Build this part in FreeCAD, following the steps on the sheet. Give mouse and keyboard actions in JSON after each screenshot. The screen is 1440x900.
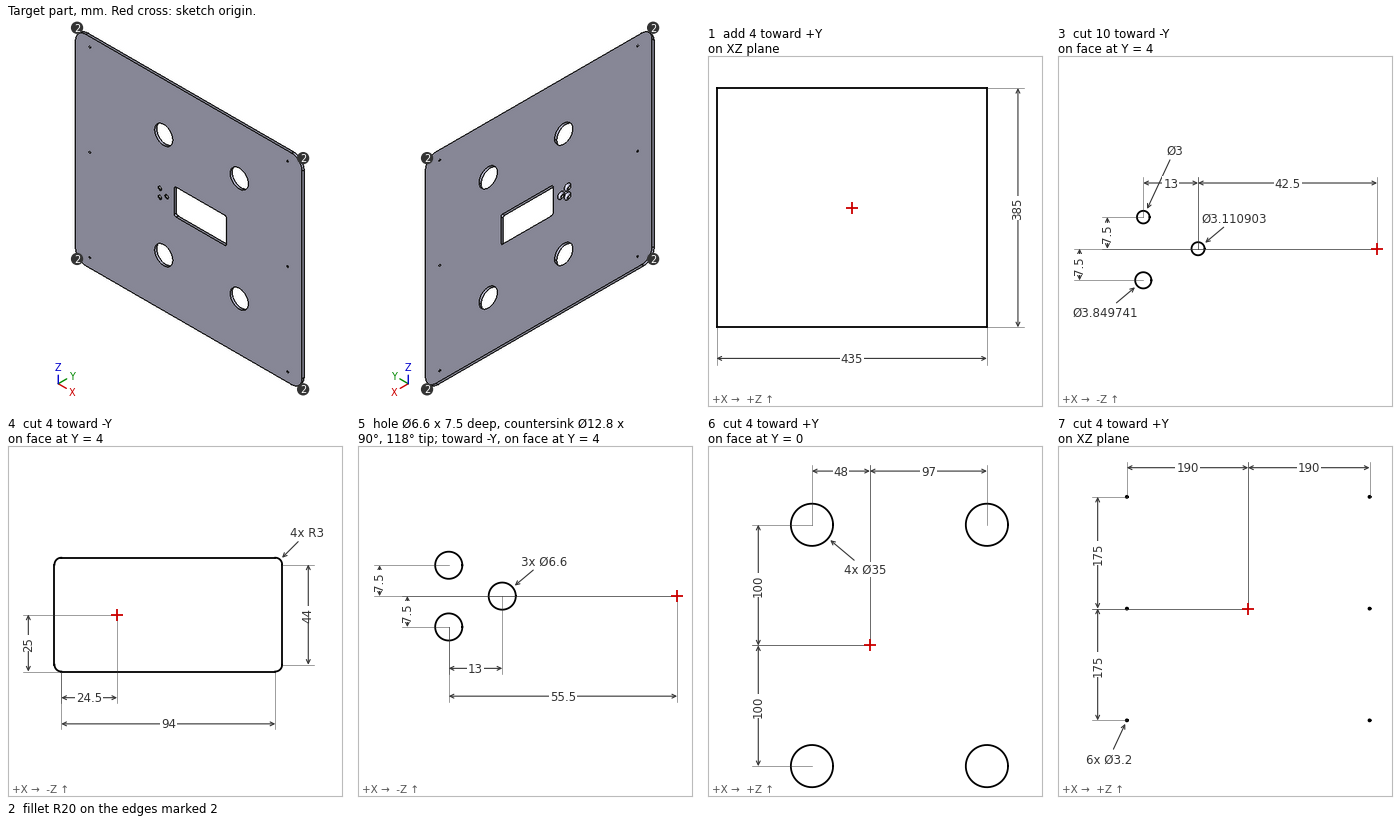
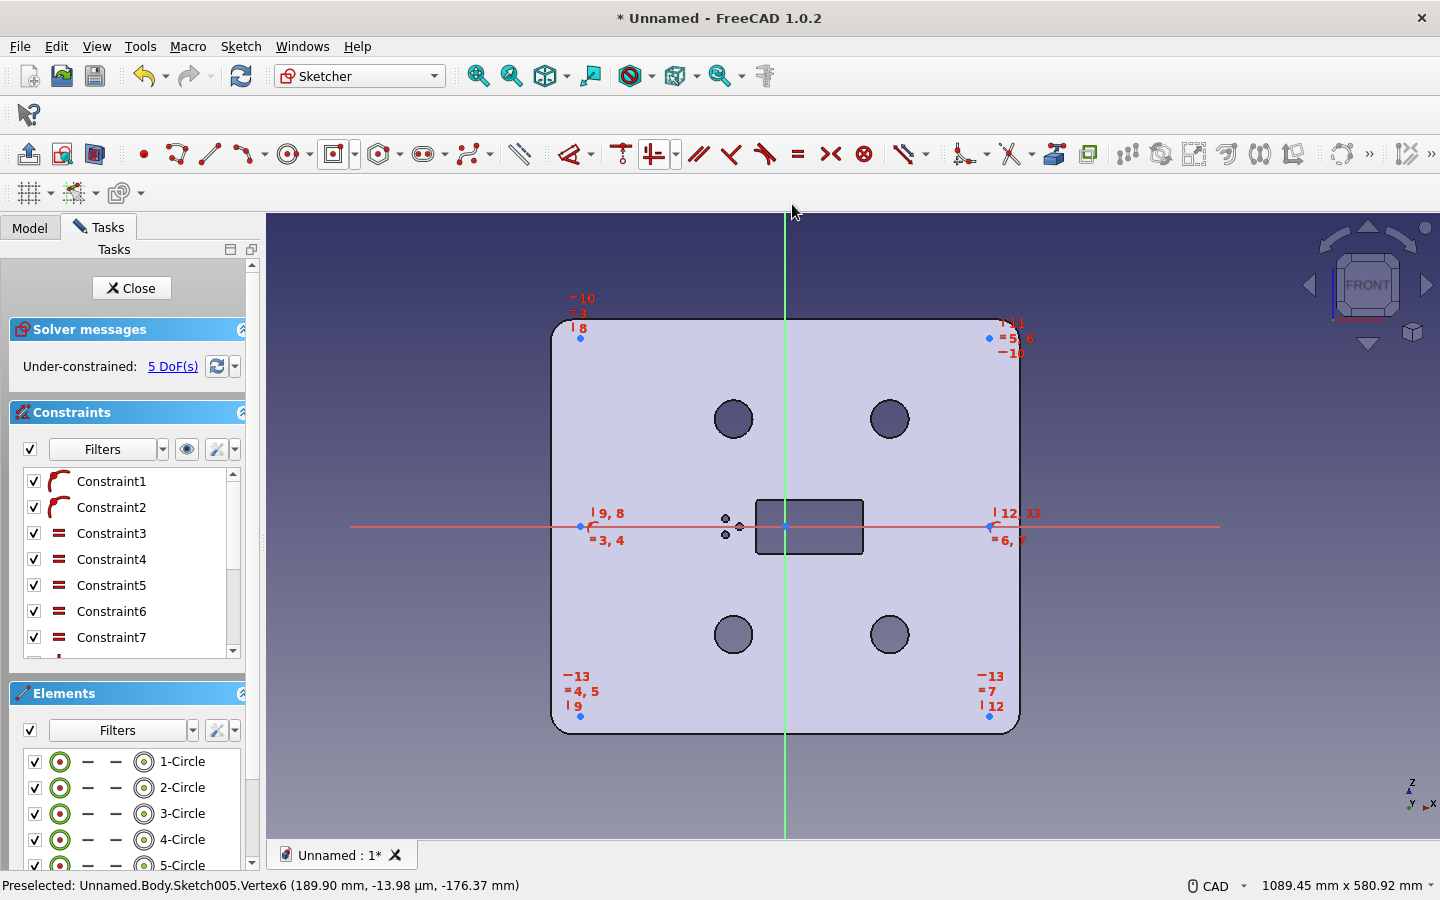
{"action": "left_click", "coordinate": [568, 154]}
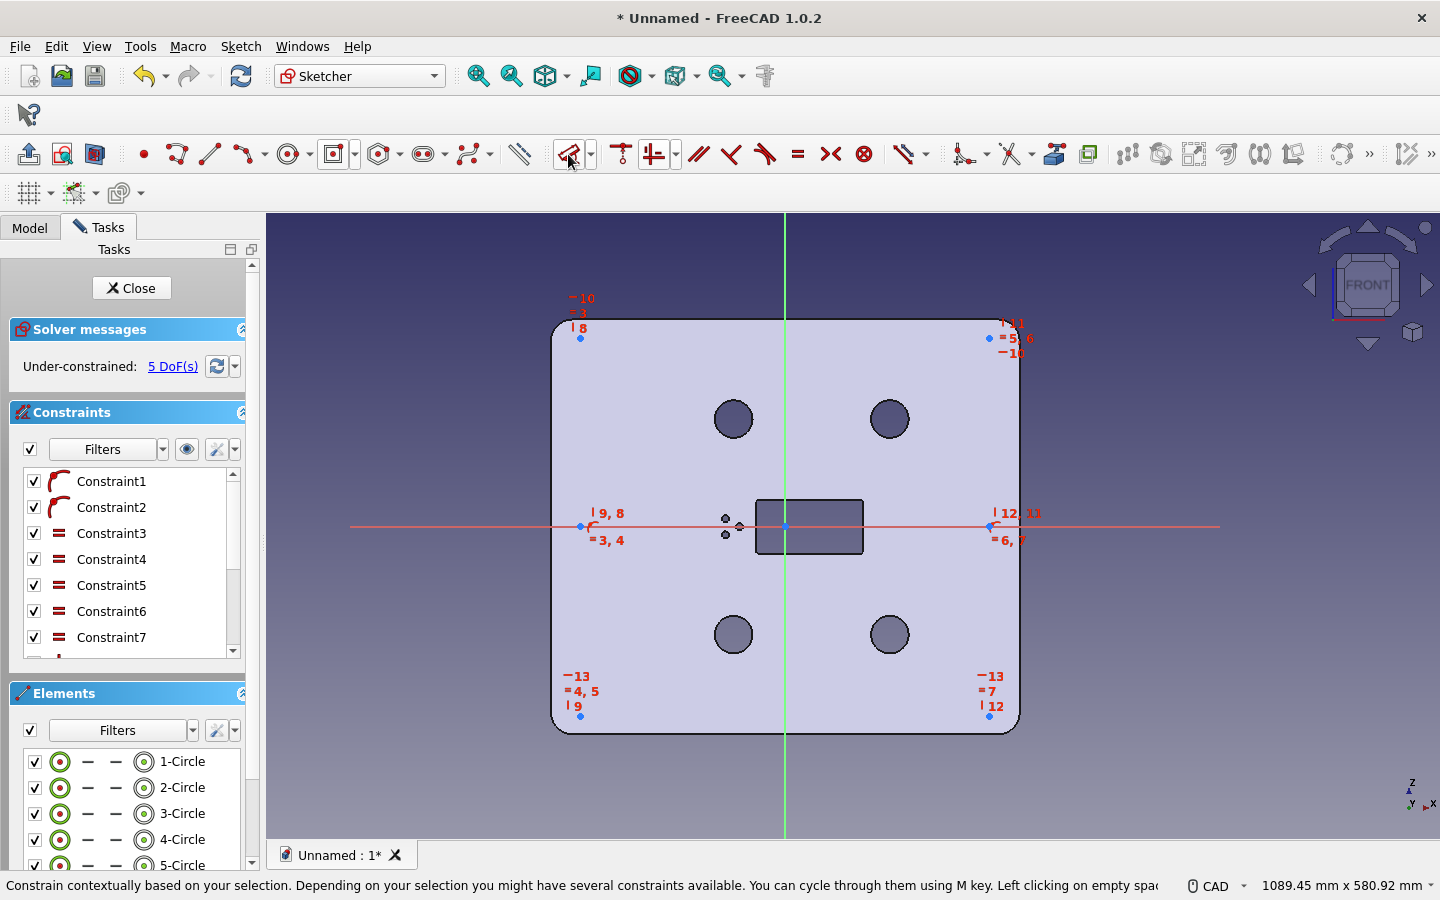
{"action": "scroll", "coordinate": [582, 337], "scroll_direction": "up", "scroll_amount": 13}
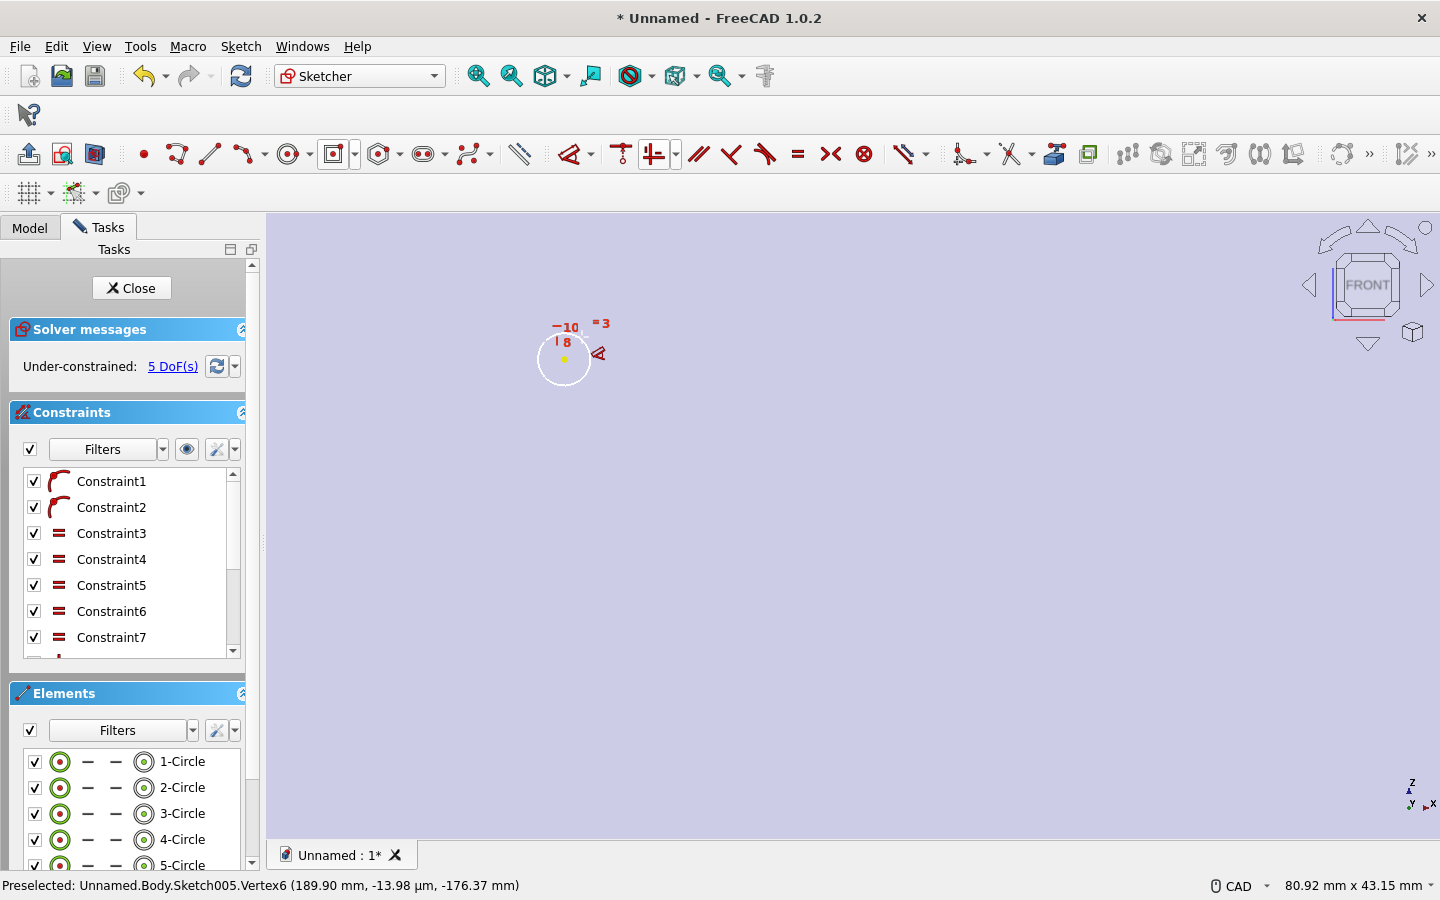
{"action": "left_click", "coordinate": [583, 341]}
{"action": "left_click", "coordinate": [606, 319]}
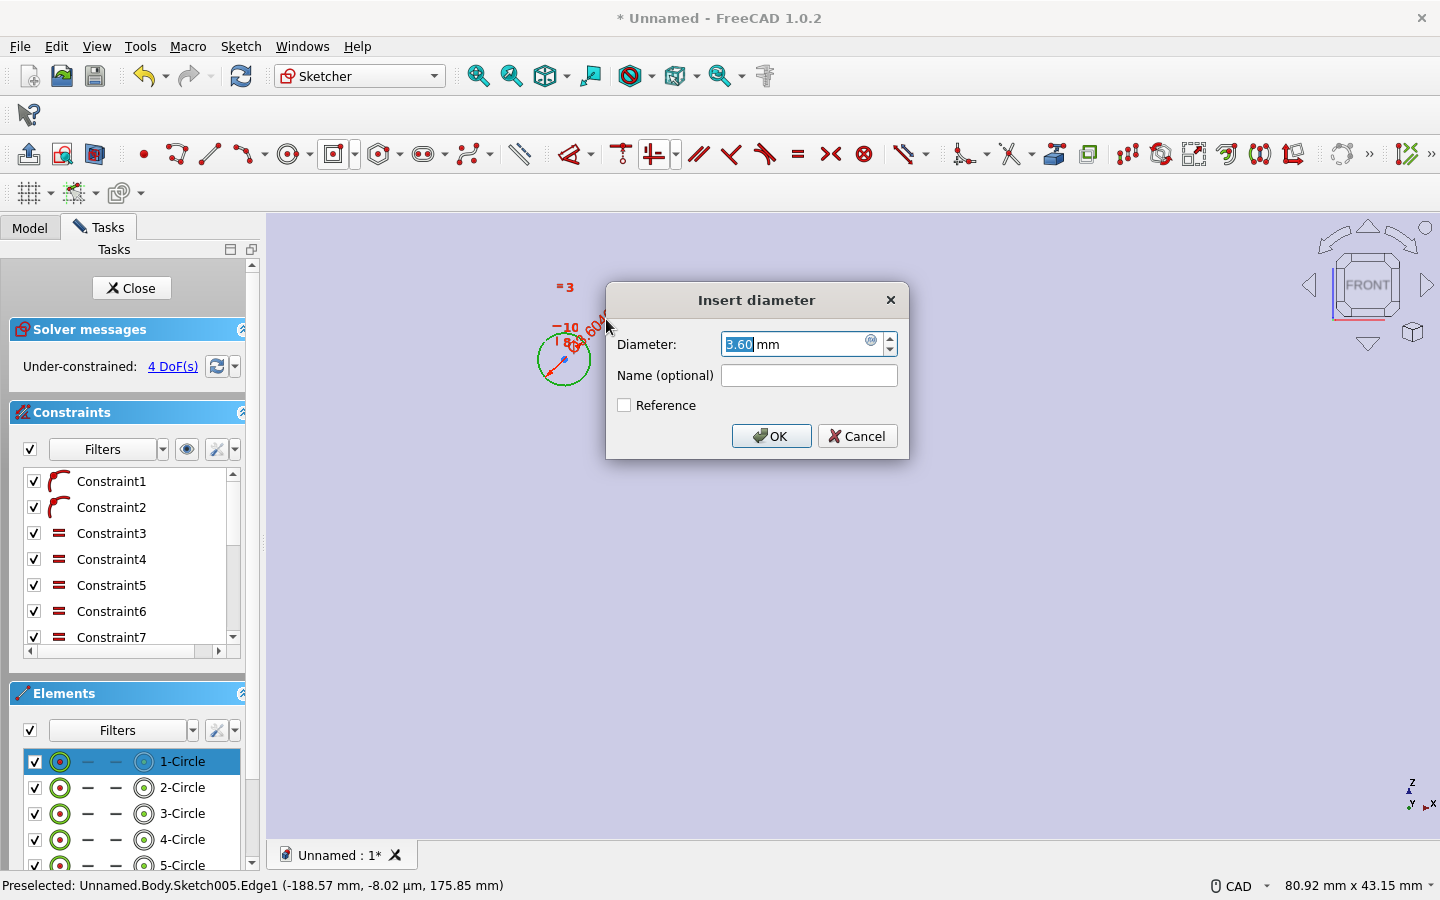
{"action": "type", "text": "3.2"}
{"action": "key", "text": "Return"}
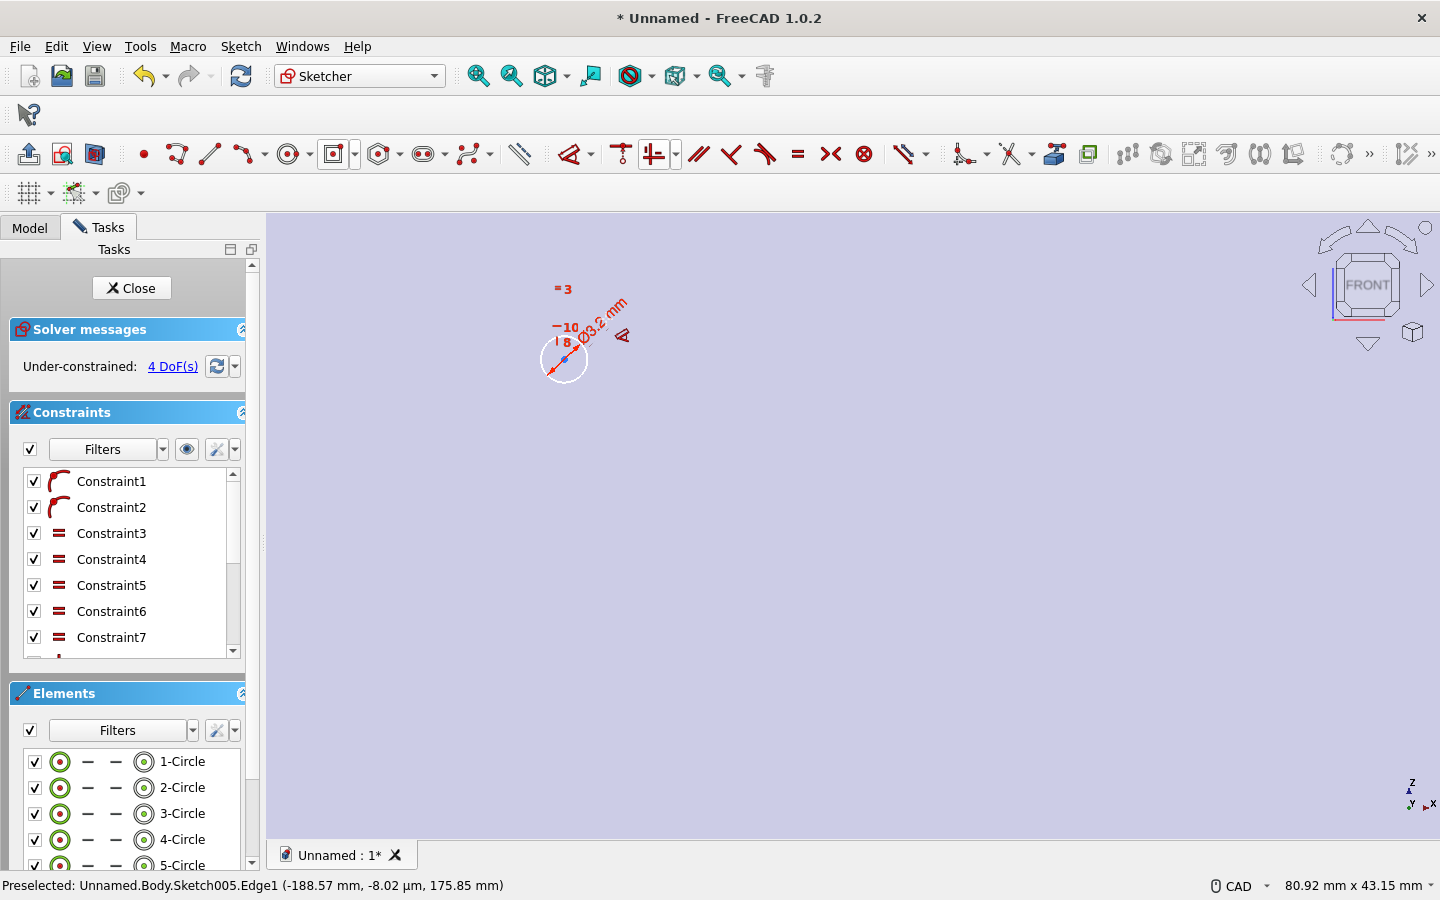
{"action": "scroll", "coordinate": [581, 336], "scroll_direction": "down", "scroll_amount": 13}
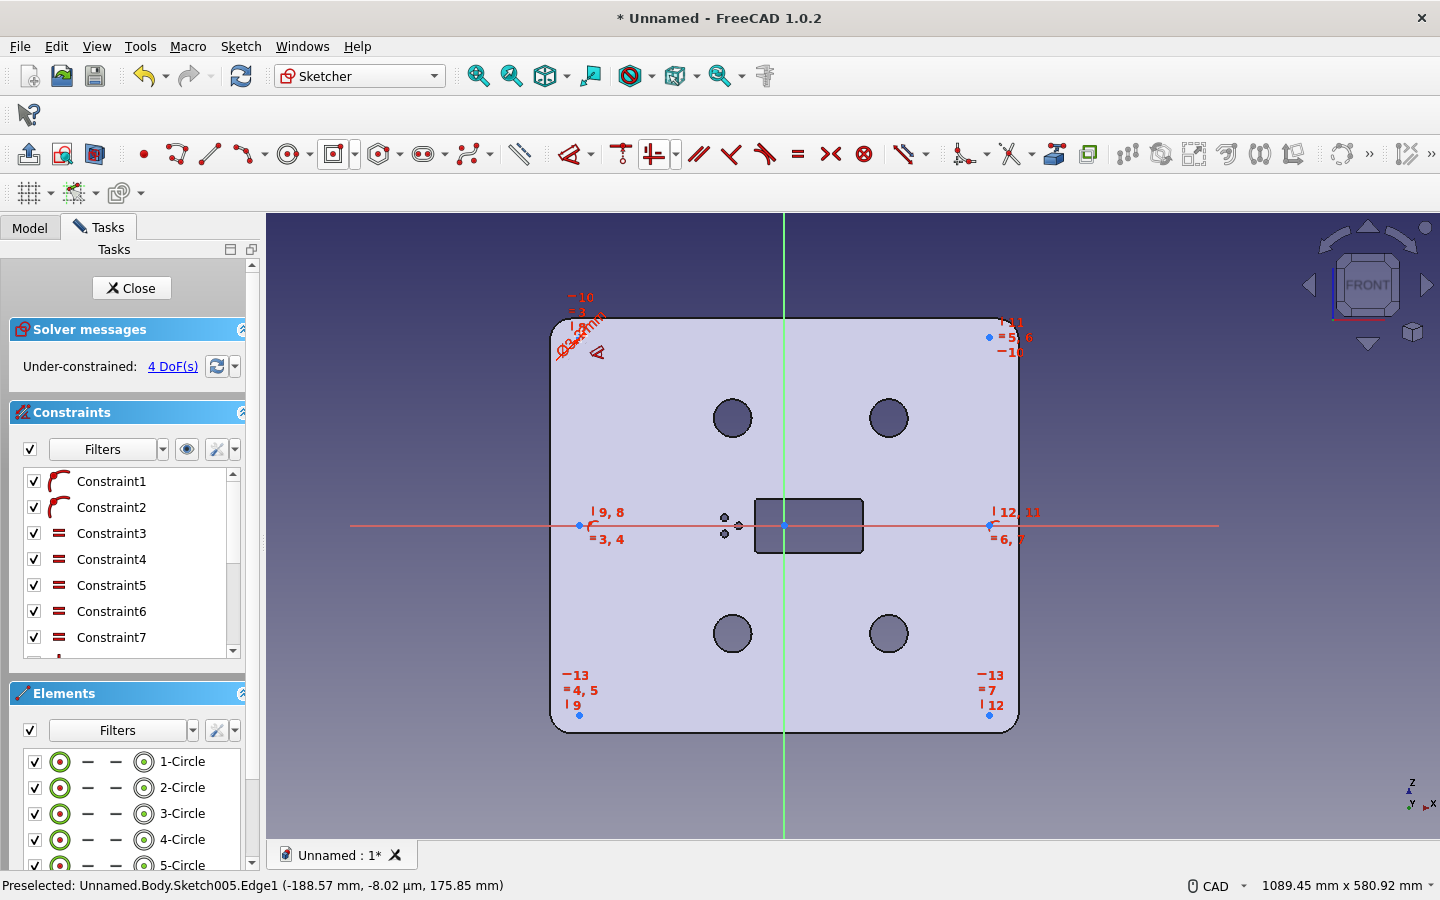
{"action": "left_click", "coordinate": [580, 338]}
{"action": "left_click", "coordinate": [682, 304]}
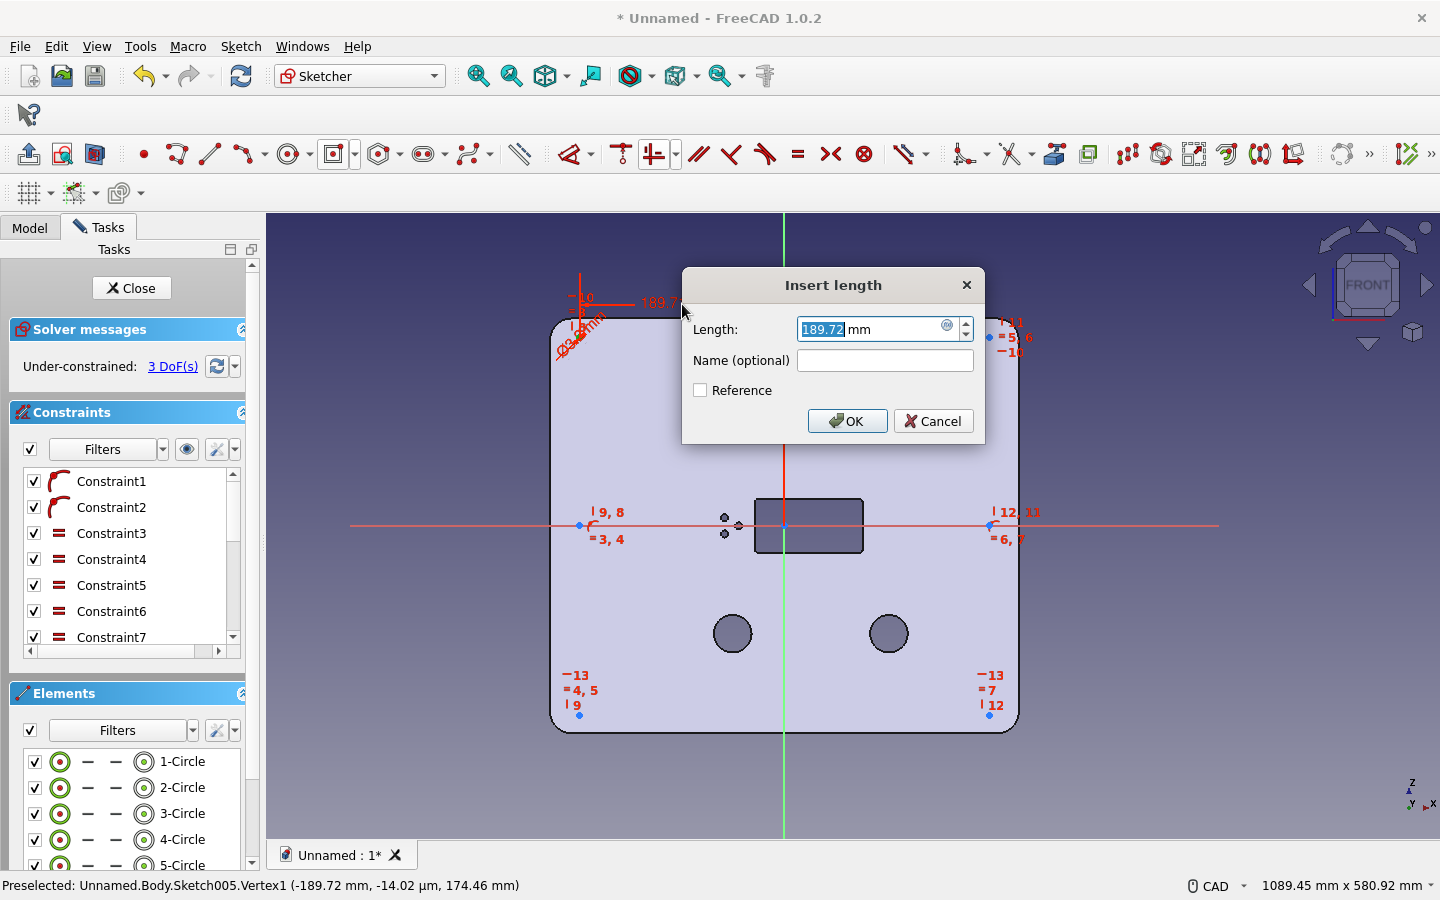
{"action": "type", "text": "190"}
{"action": "key", "text": "Return"}